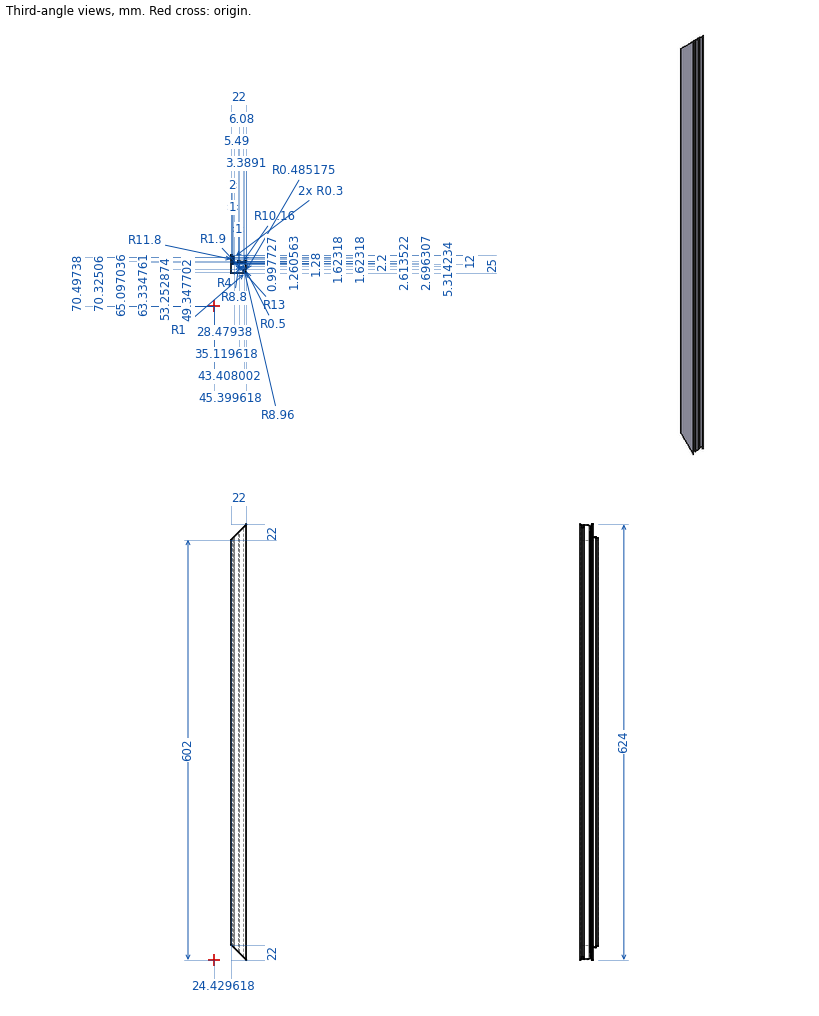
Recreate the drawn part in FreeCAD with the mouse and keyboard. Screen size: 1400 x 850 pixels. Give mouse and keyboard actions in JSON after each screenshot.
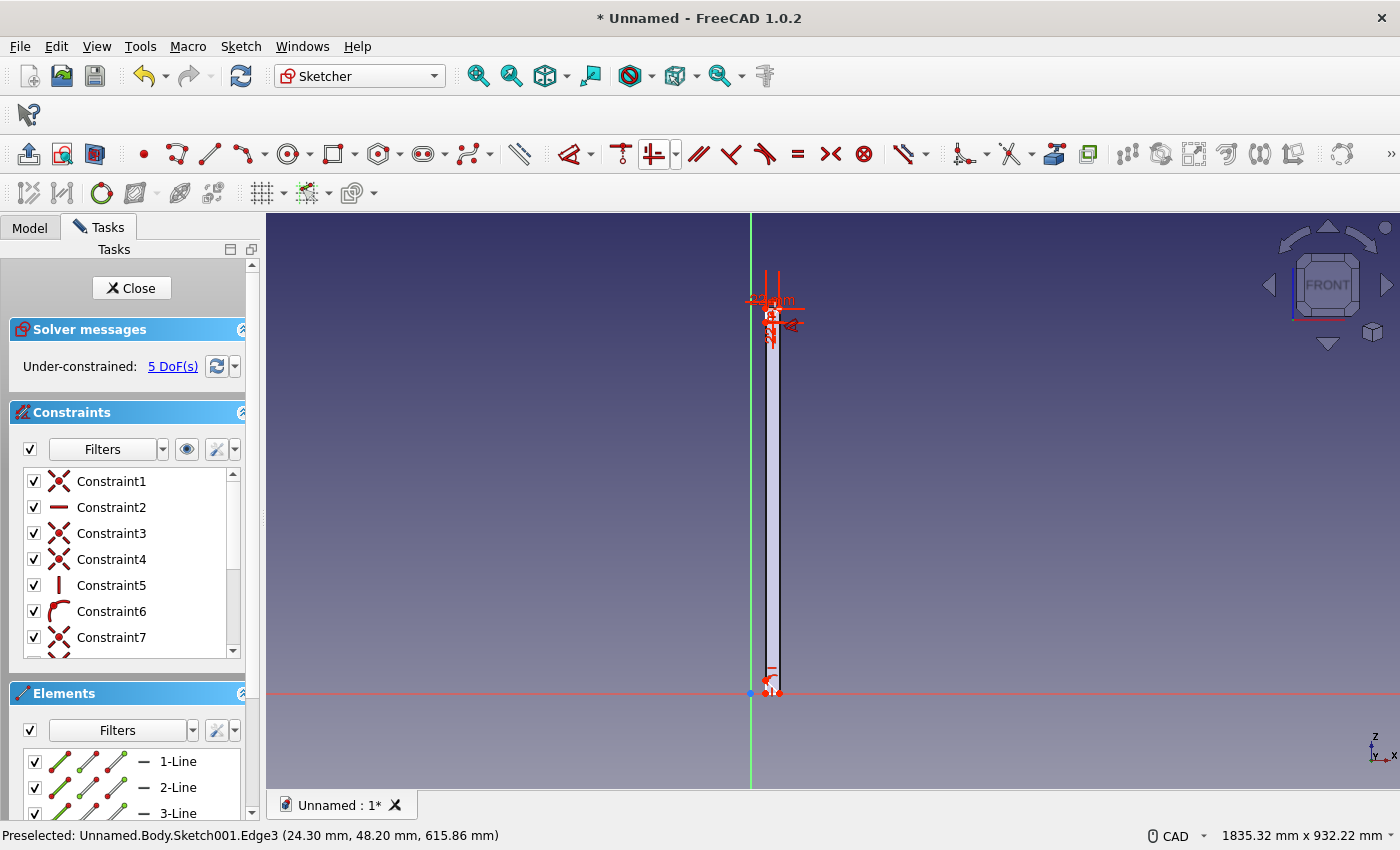
{"action": "scroll", "coordinate": [770, 694], "scroll_direction": "up", "scroll_amount": 6}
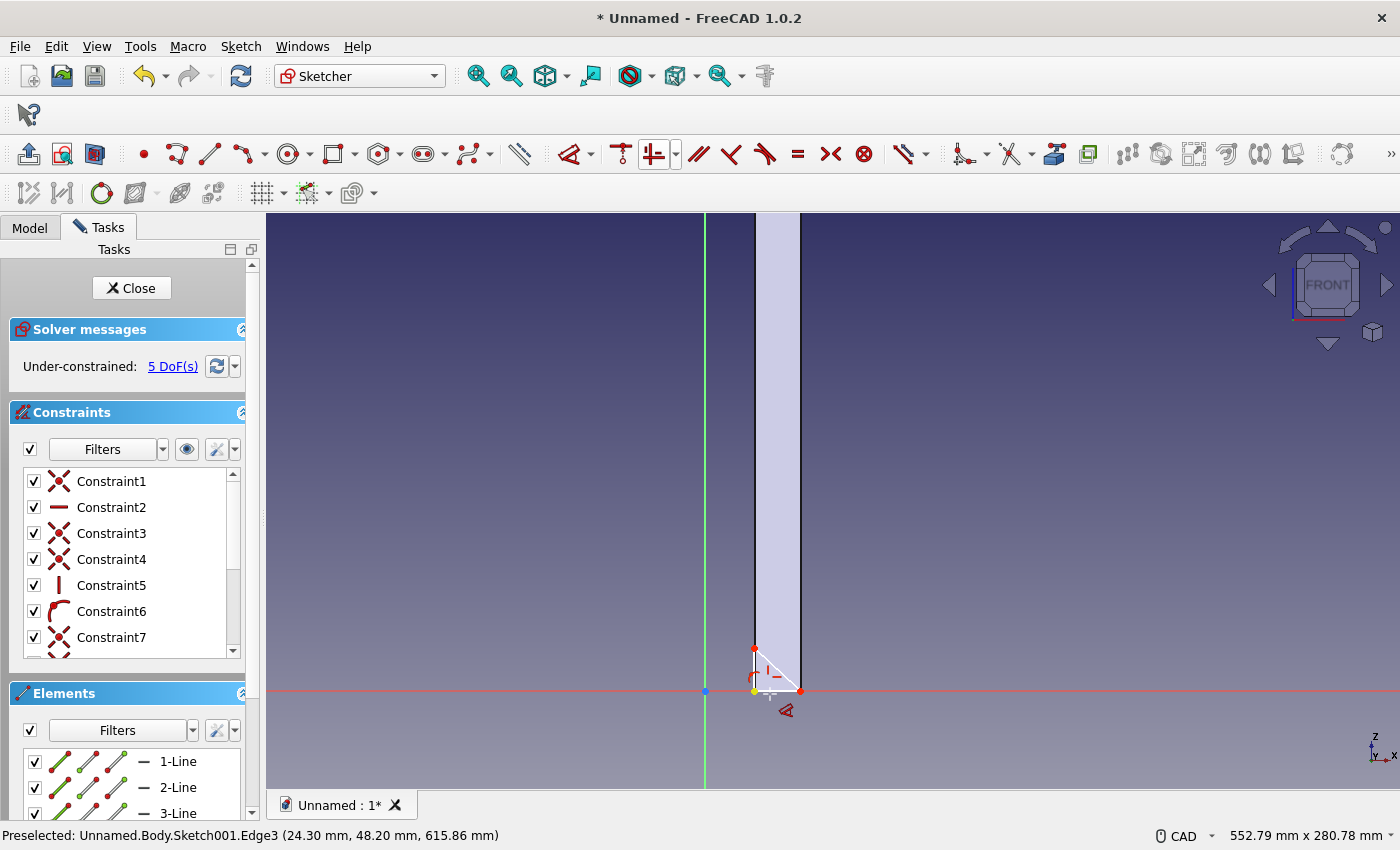
{"action": "left_click", "coordinate": [768, 691]}
{"action": "left_click", "coordinate": [778, 725]}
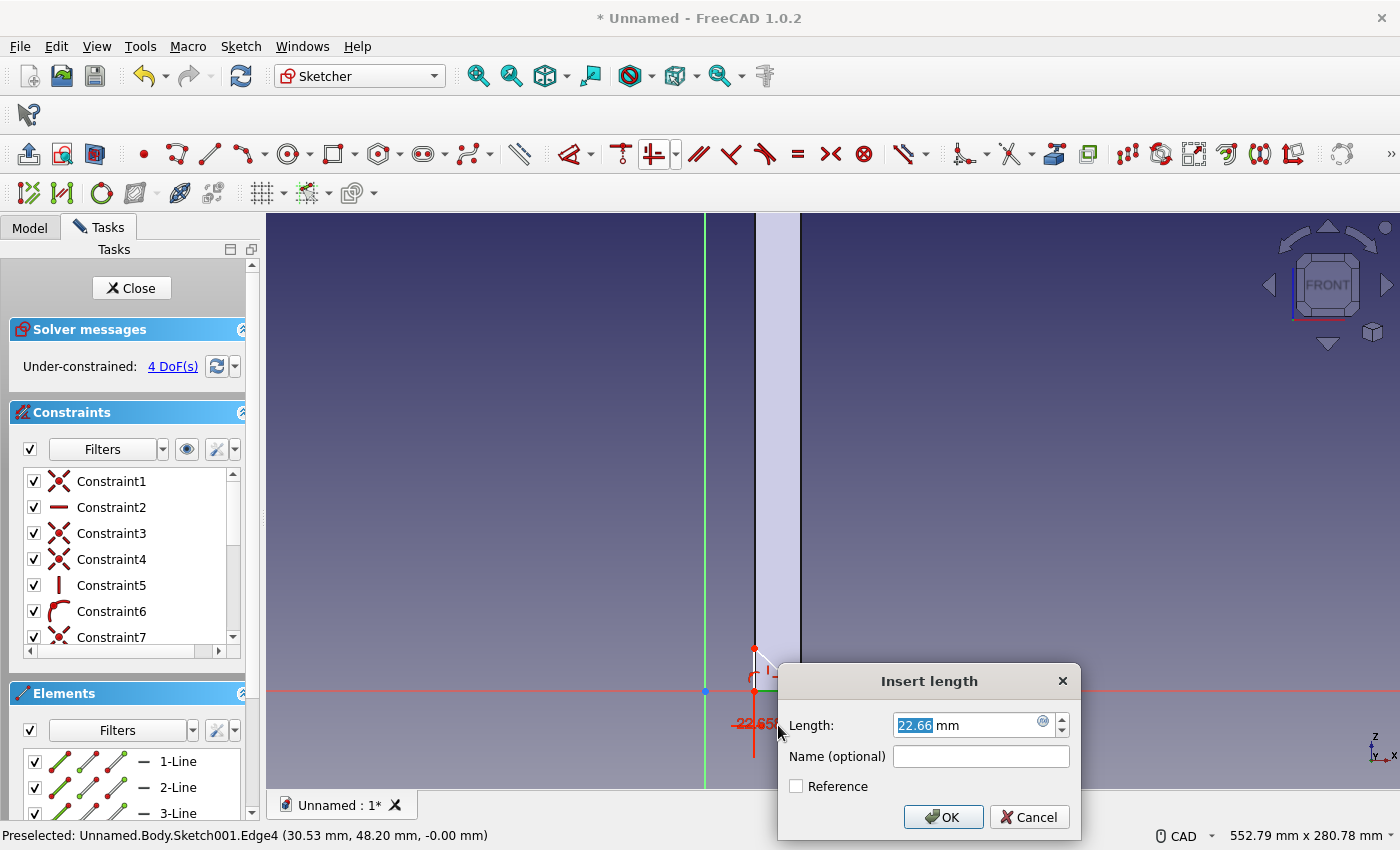
{"action": "type", "text": "22"}
{"action": "key", "text": "Return"}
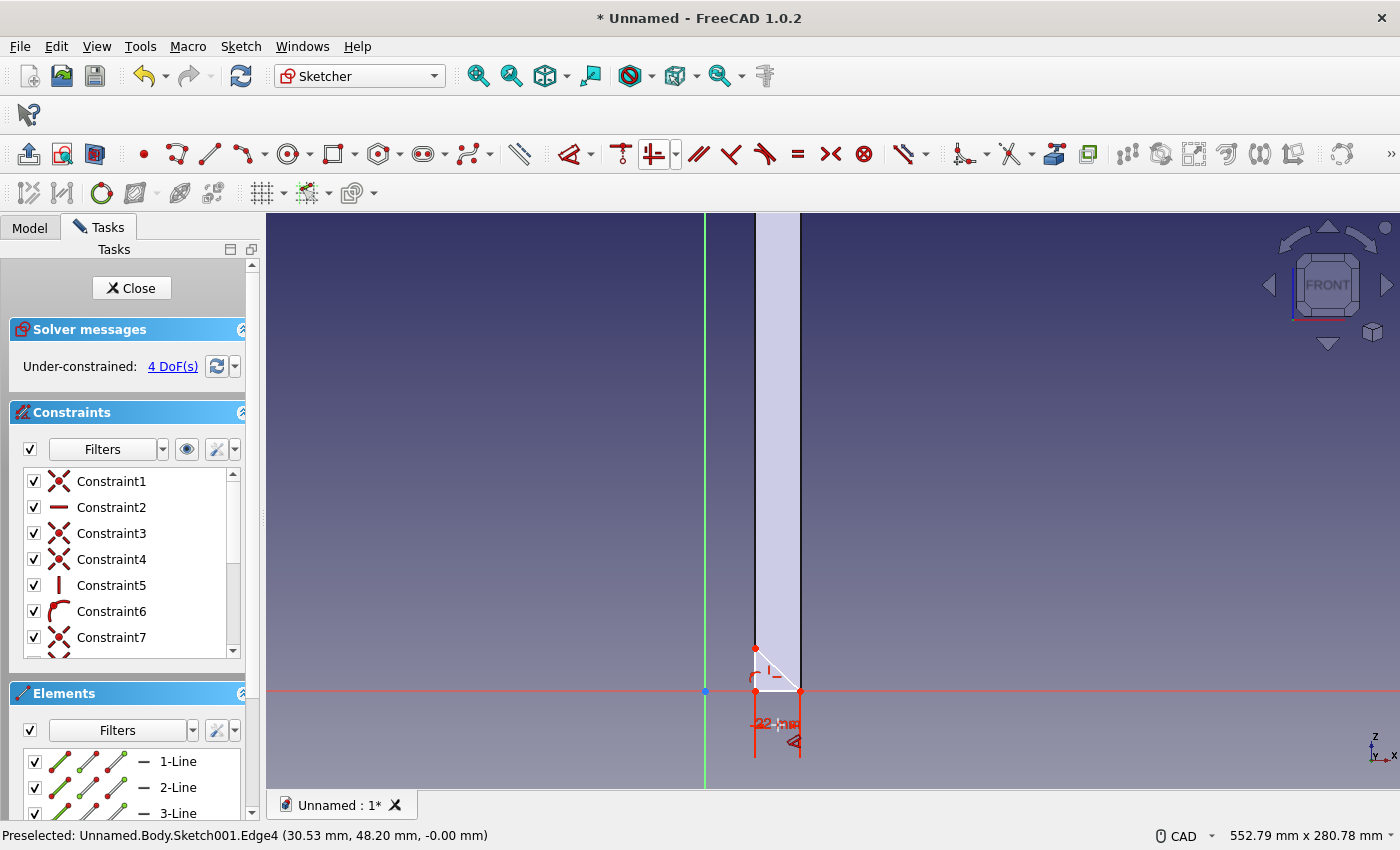
{"action": "scroll", "coordinate": [755, 661], "scroll_direction": "up", "scroll_amount": 2}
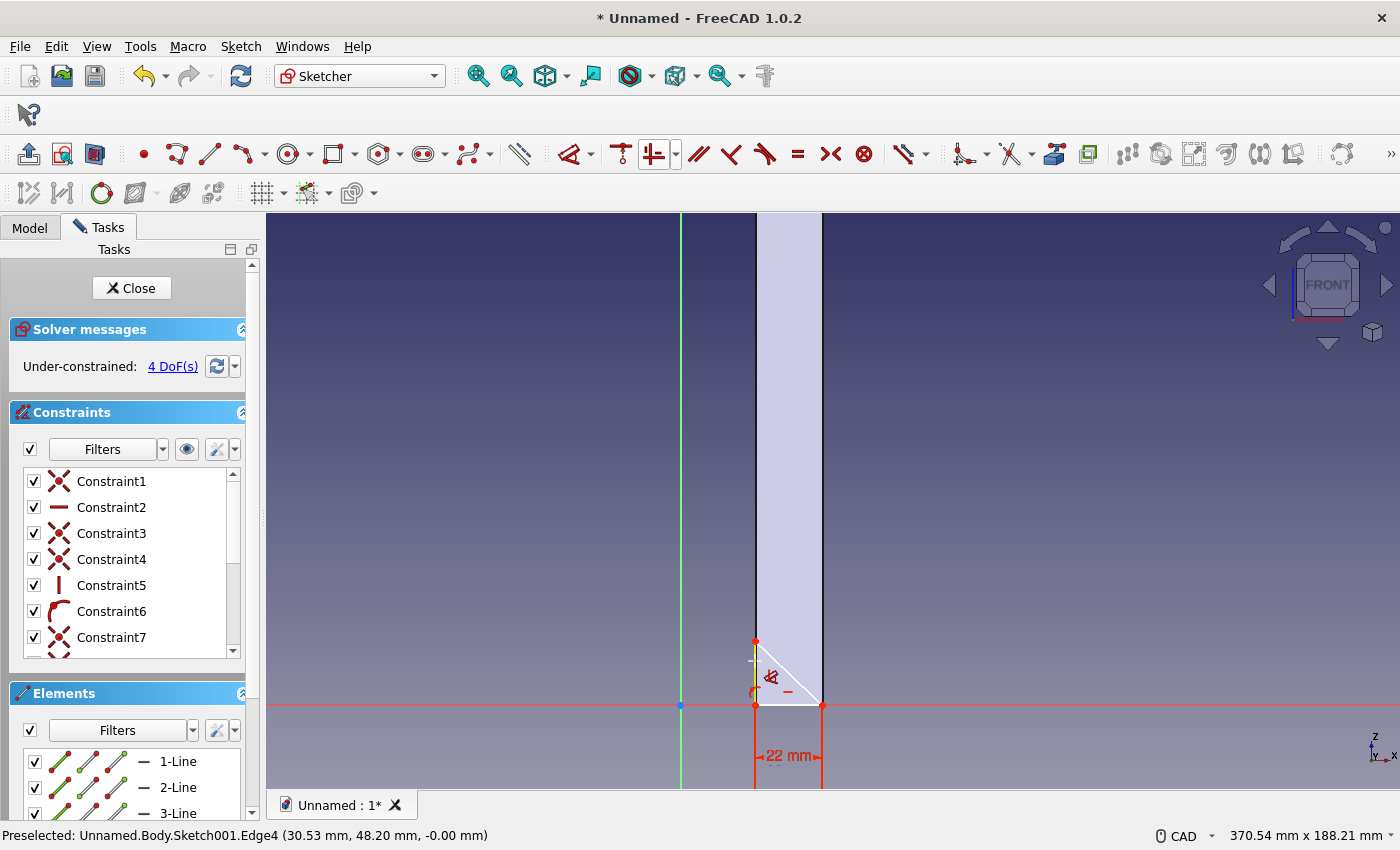
{"action": "left_click", "coordinate": [755, 661]}
{"action": "left_click", "coordinate": [789, 651]}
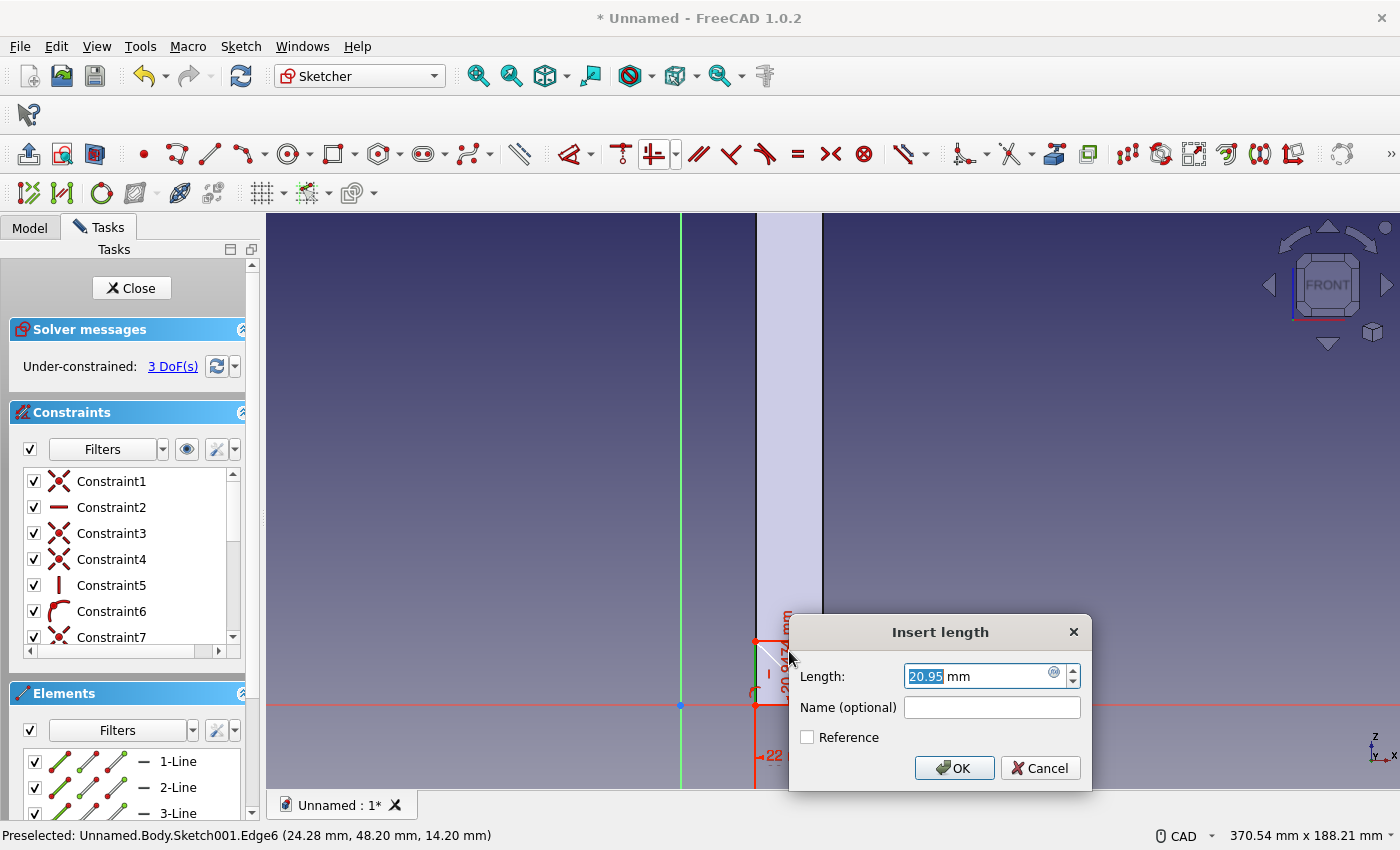
{"action": "type", "text": "22"}
{"action": "key", "text": "Return"}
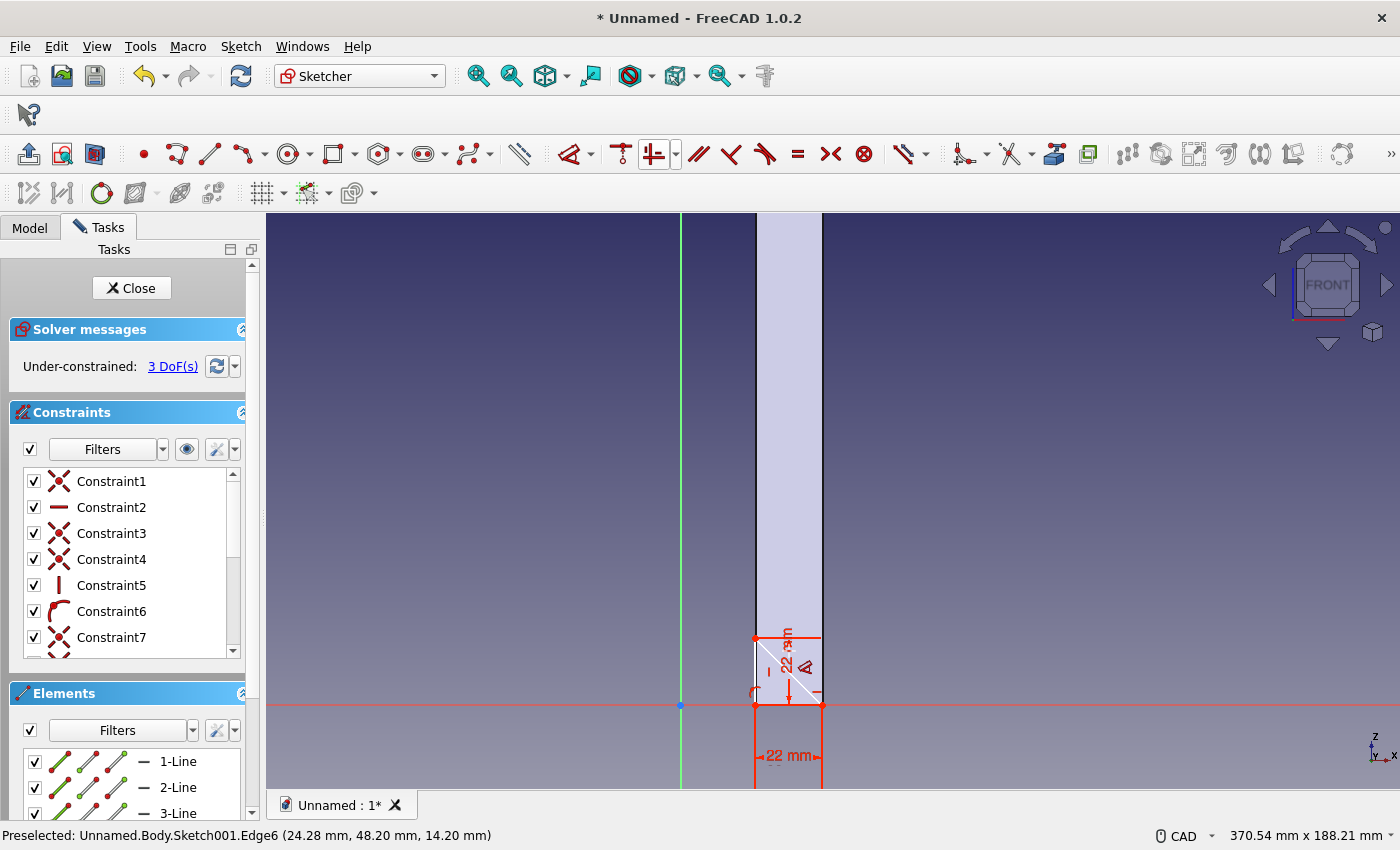
{"action": "scroll", "coordinate": [768, 691], "scroll_direction": "down", "scroll_amount": 8}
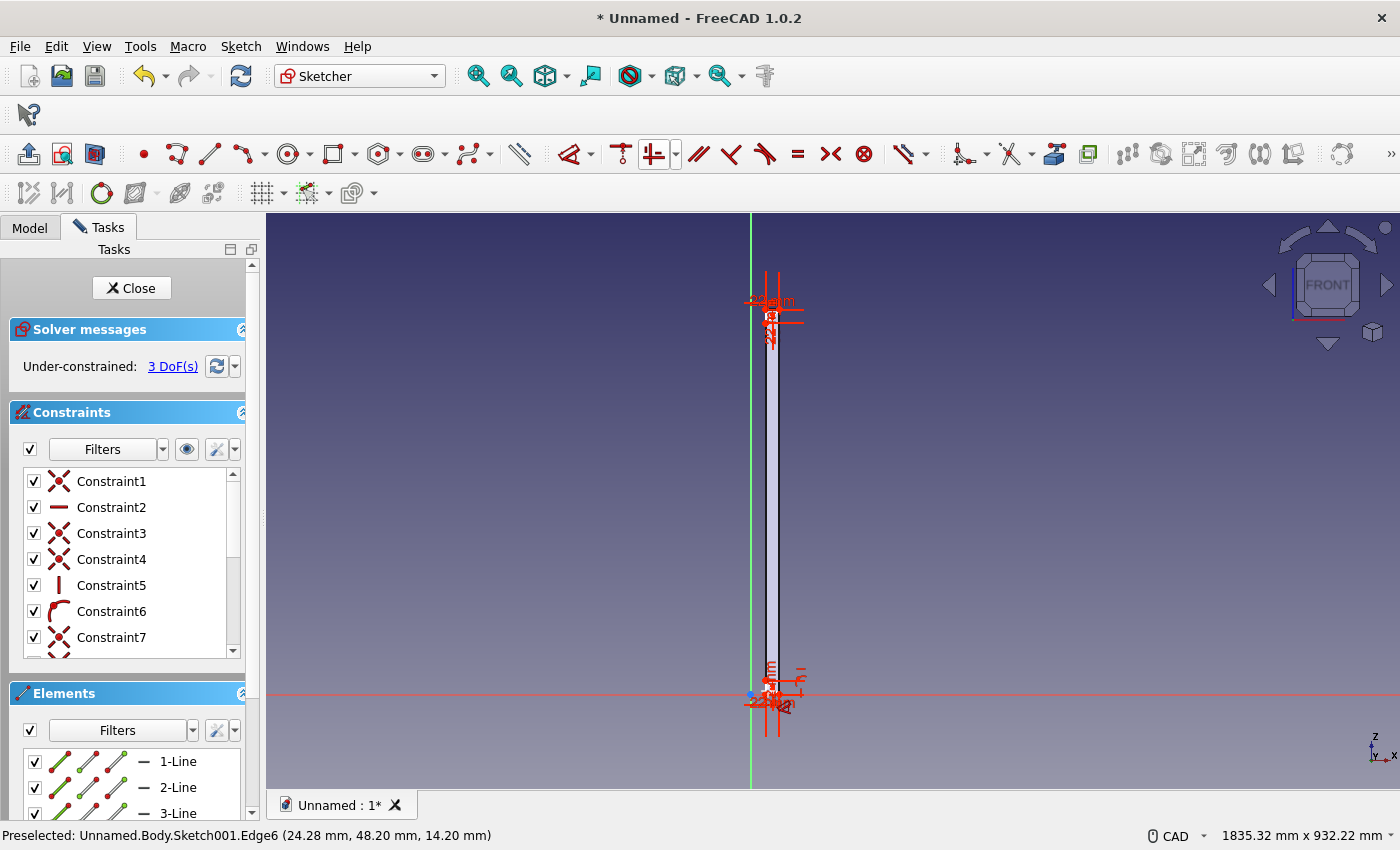
{"action": "left_click", "coordinate": [766, 323]}
{"action": "left_click", "coordinate": [717, 509]}